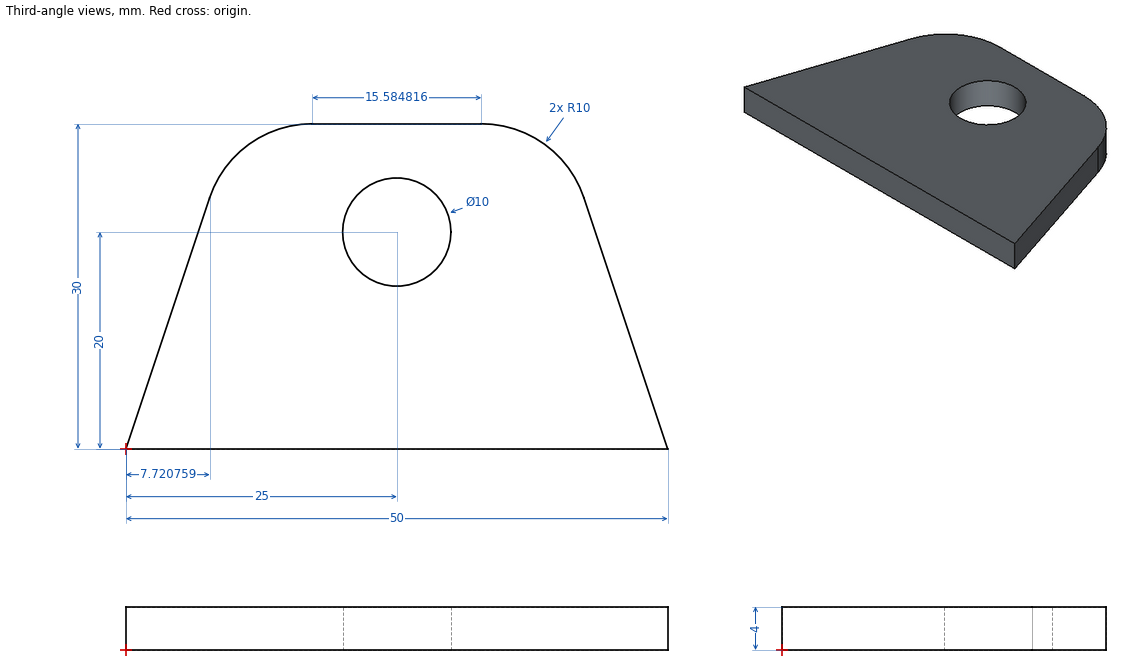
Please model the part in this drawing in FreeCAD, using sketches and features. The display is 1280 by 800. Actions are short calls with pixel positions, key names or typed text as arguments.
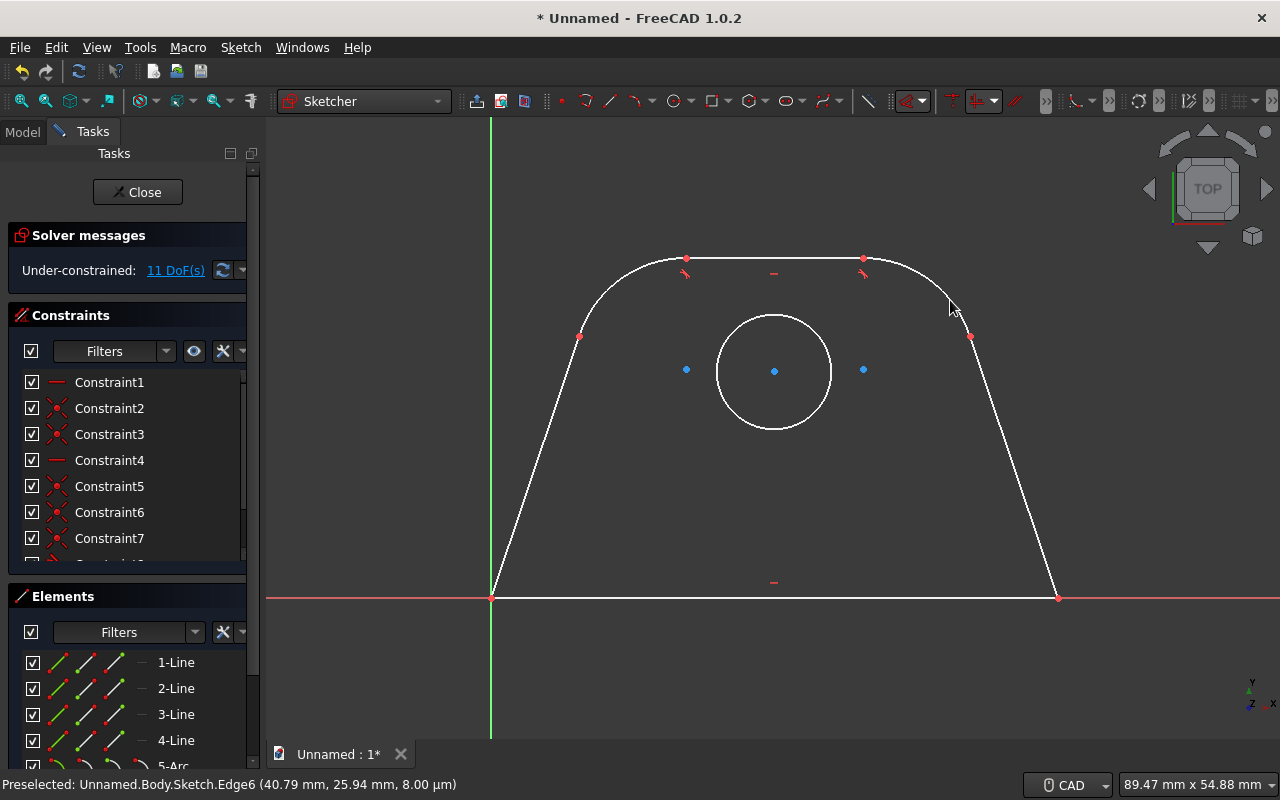
click(553, 415)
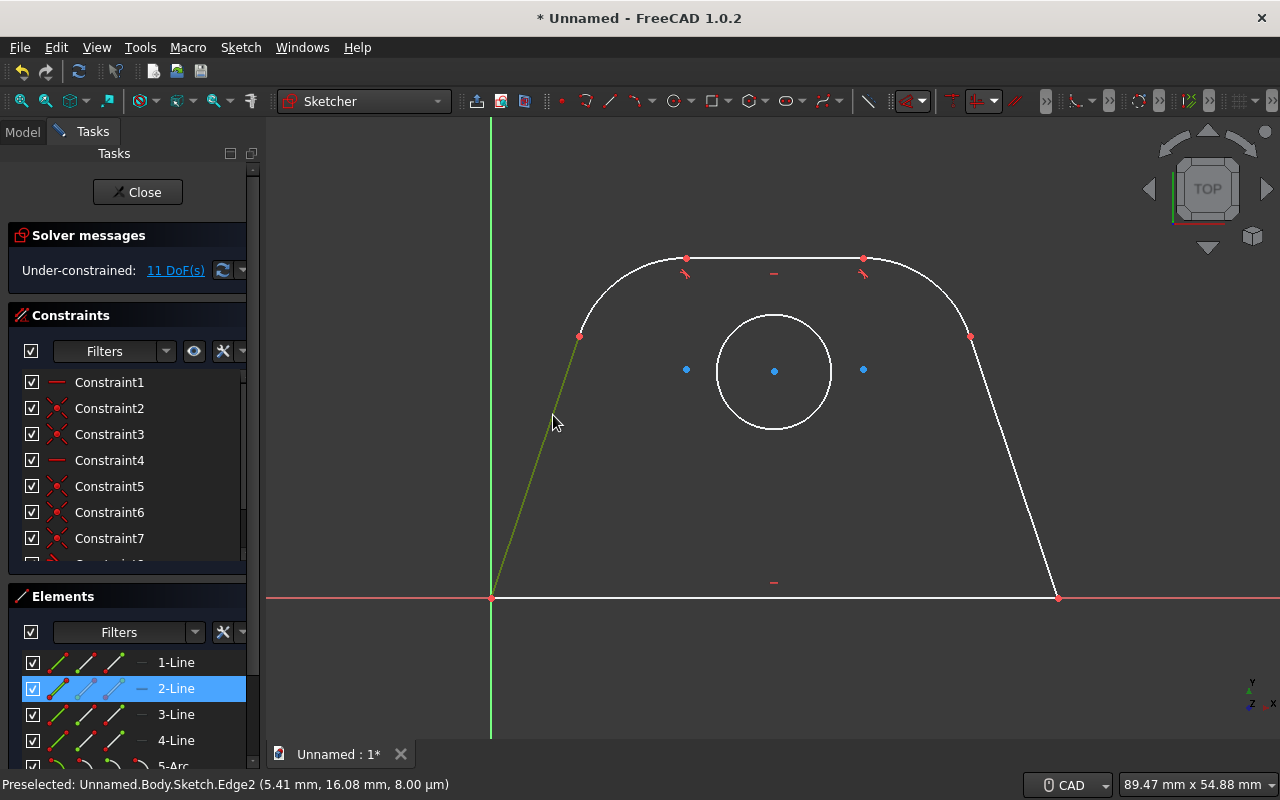
click(644, 266)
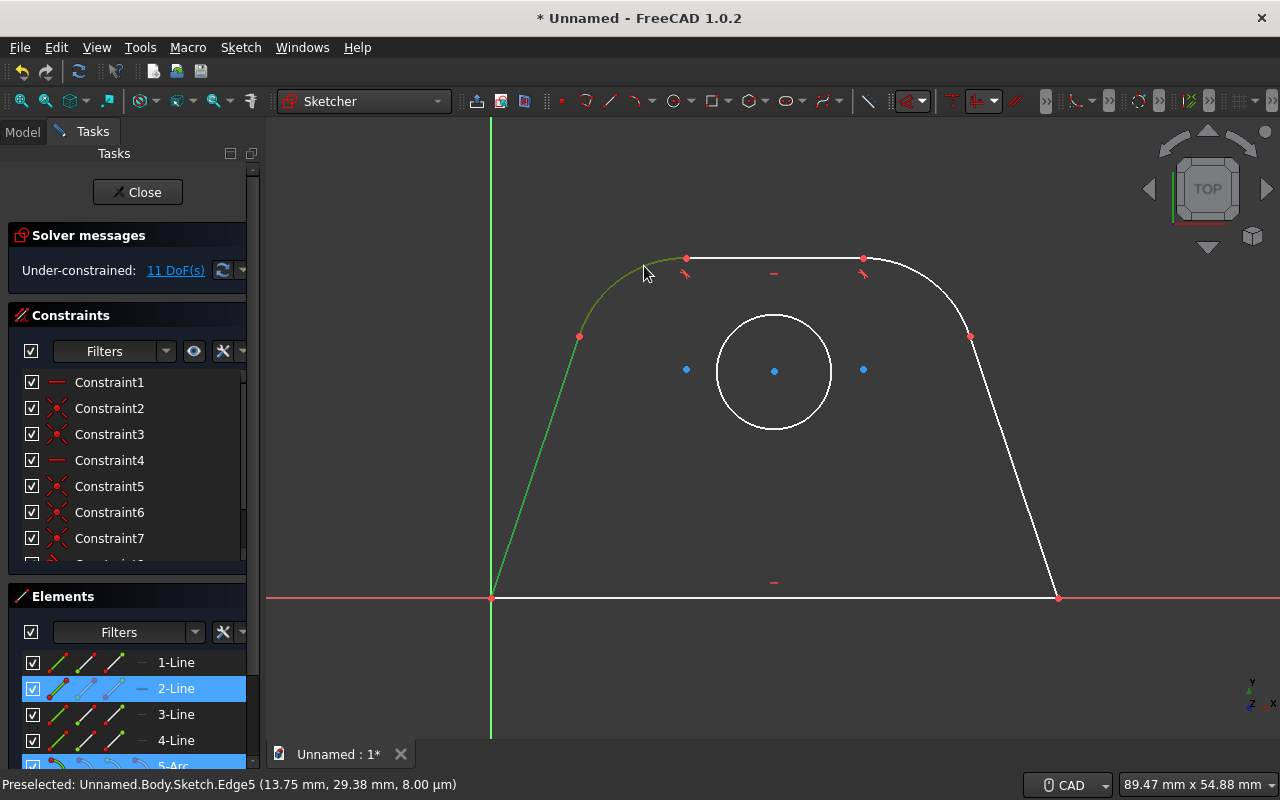
key(t)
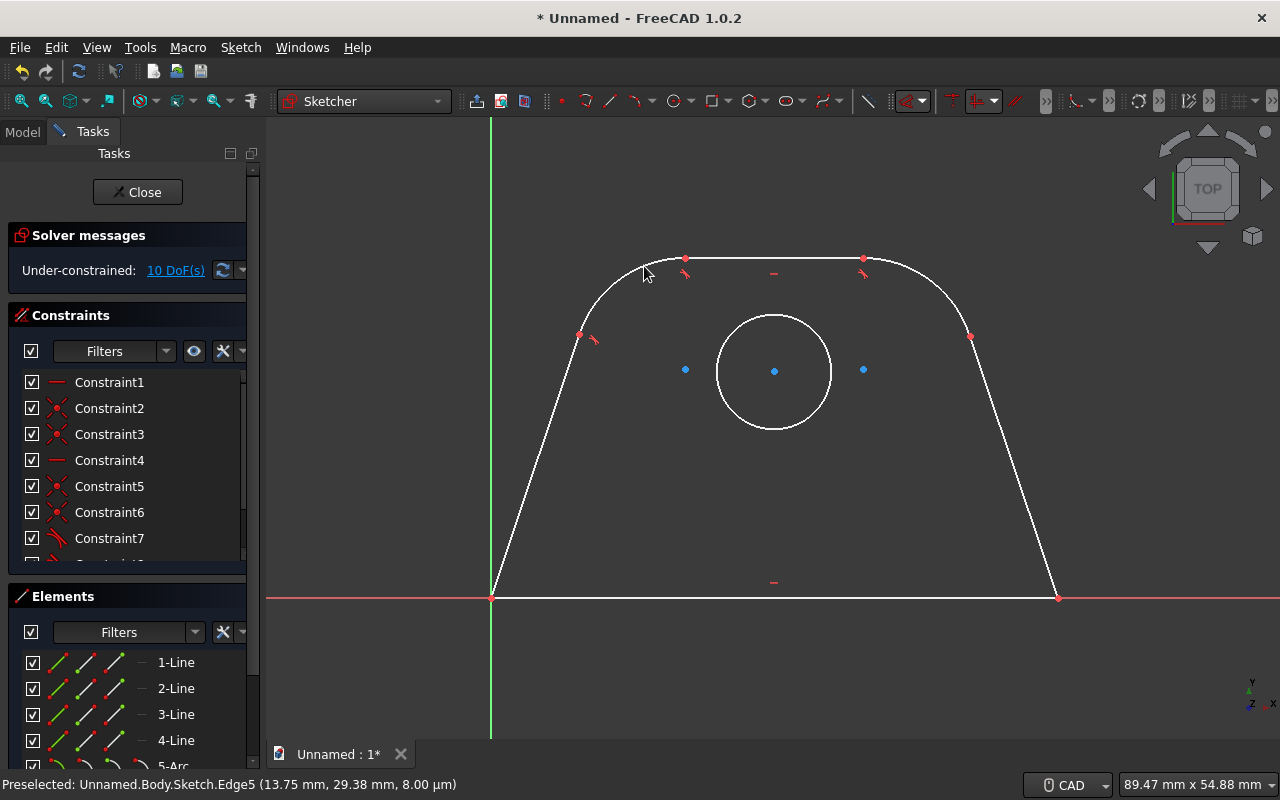
click(1032, 520)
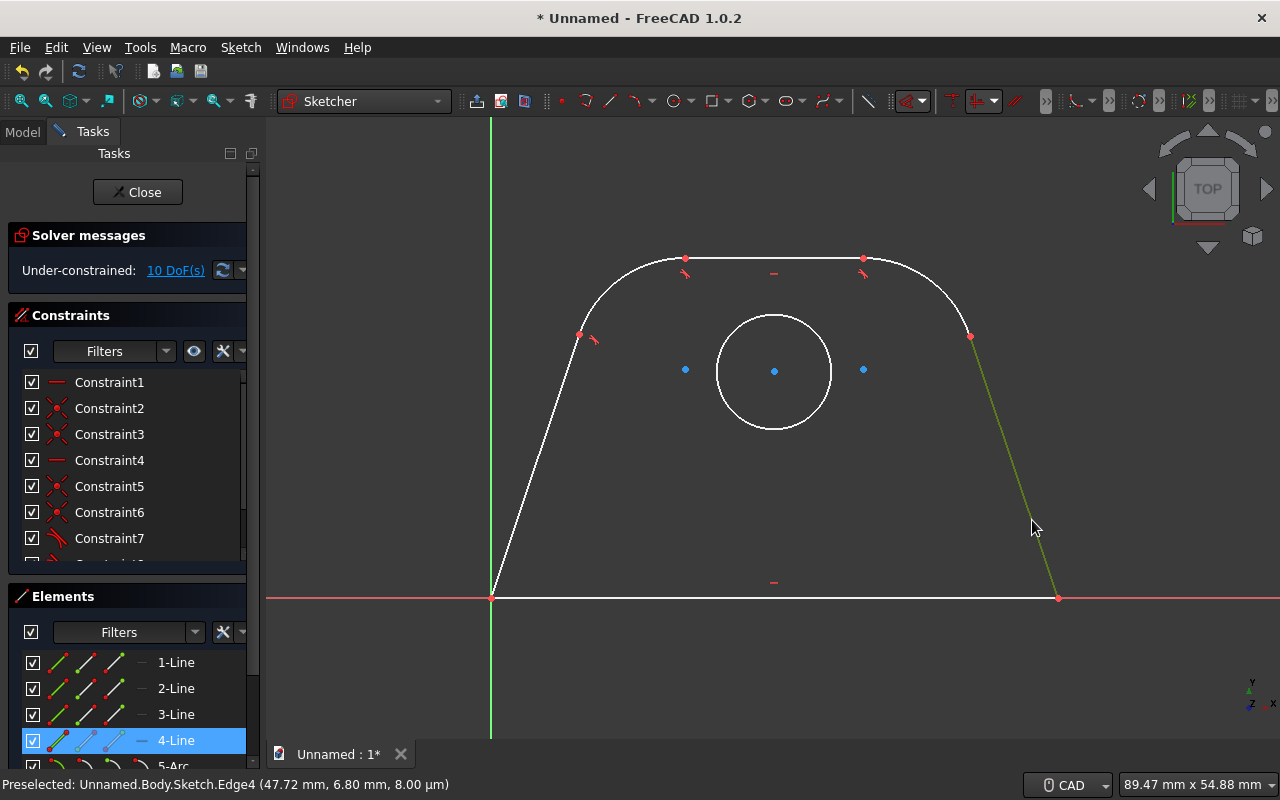
click(950, 300)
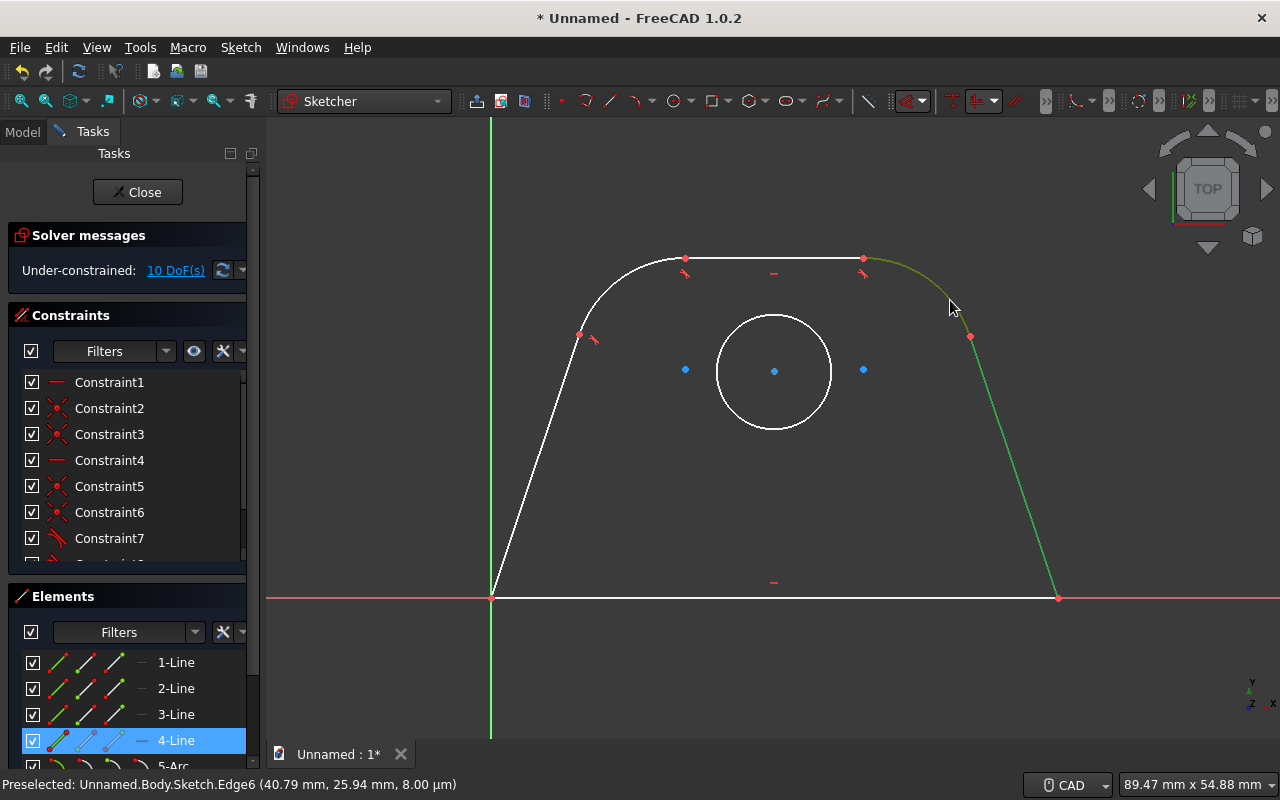
key(t)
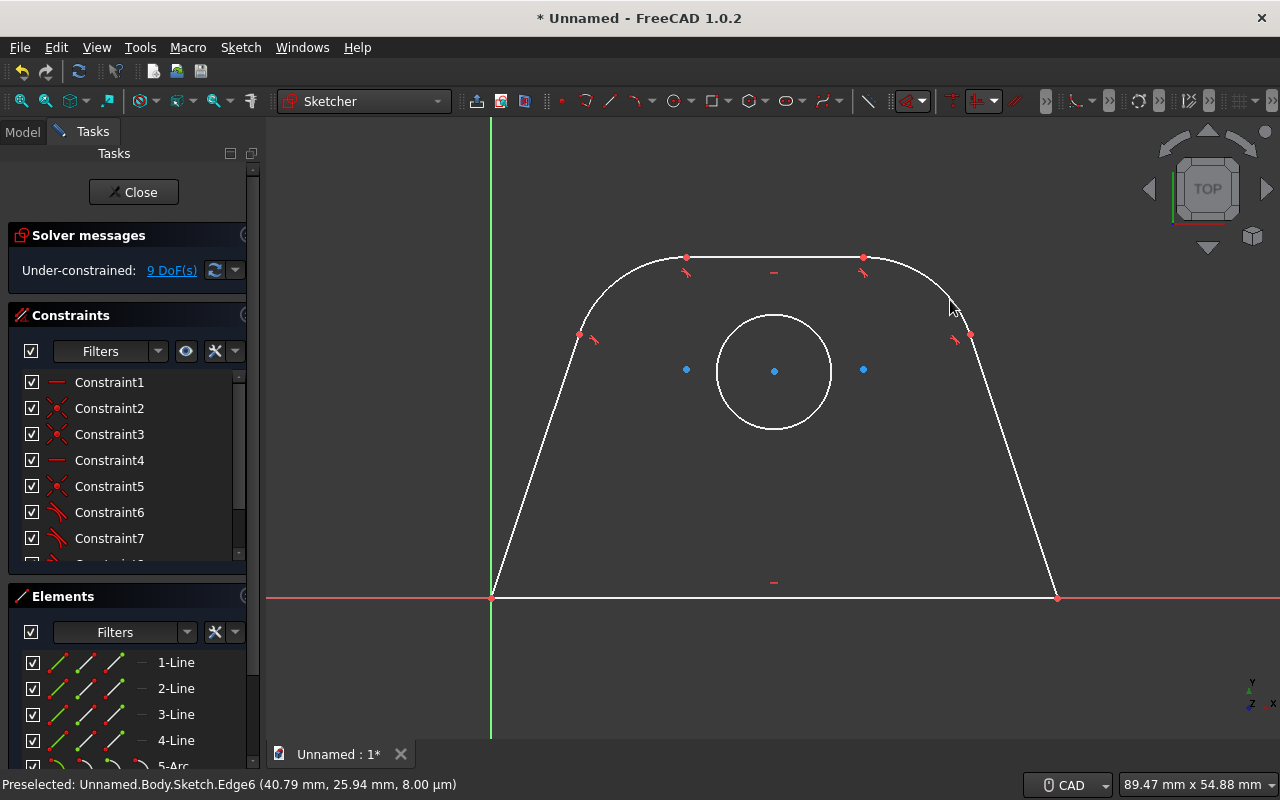
click(645, 265)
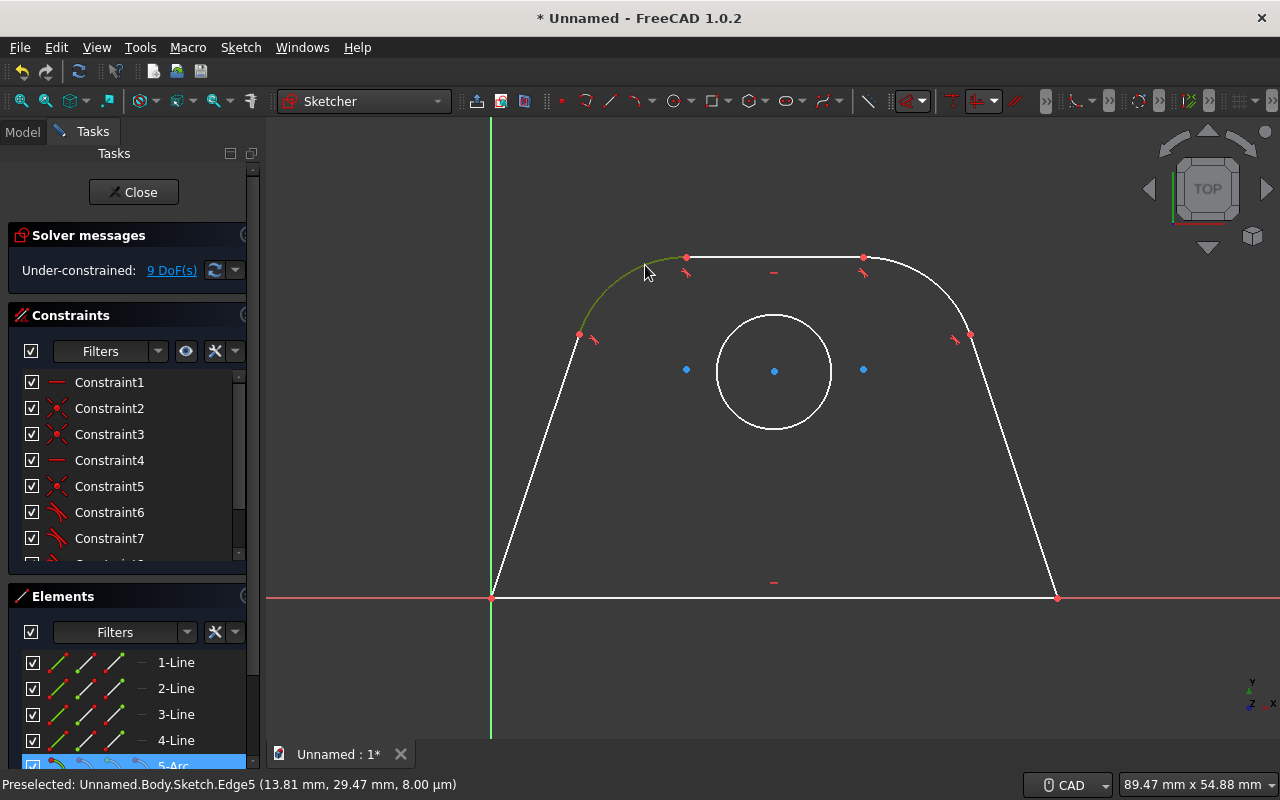
click(950, 298)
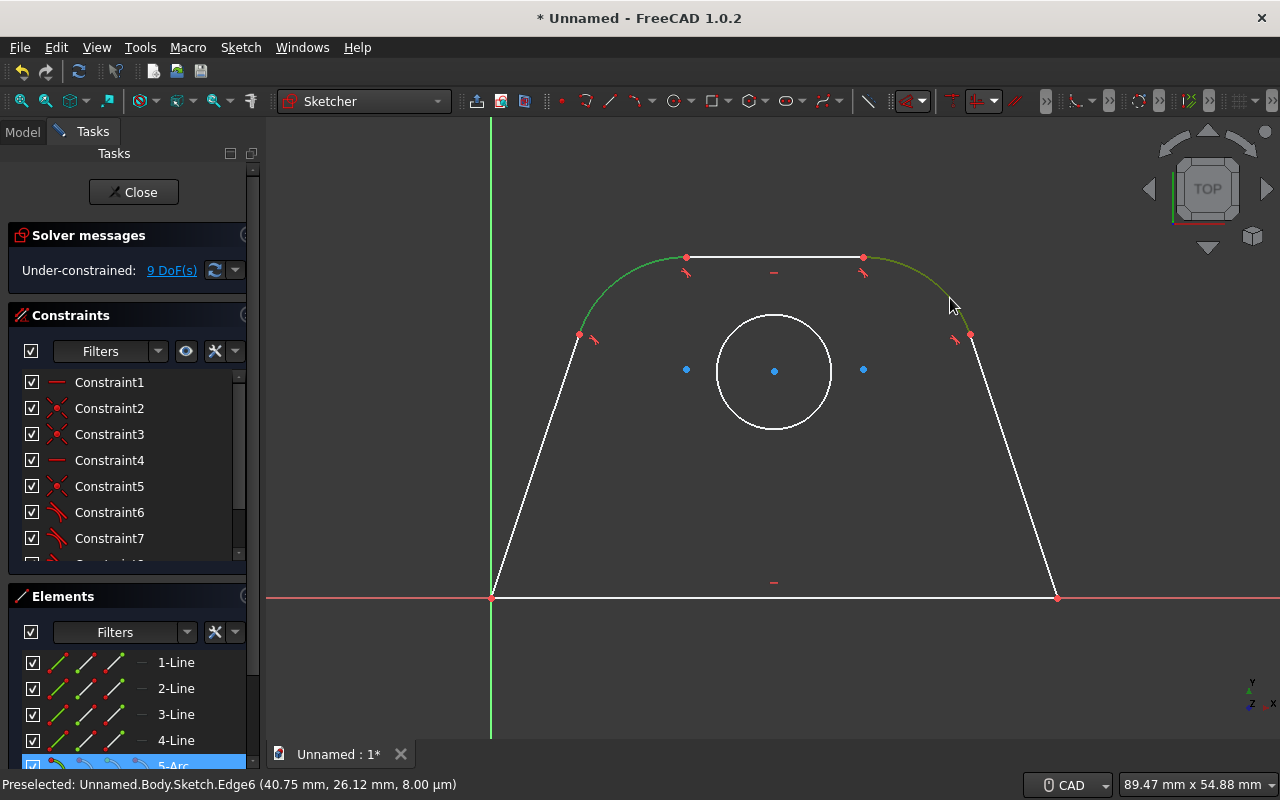
key(e)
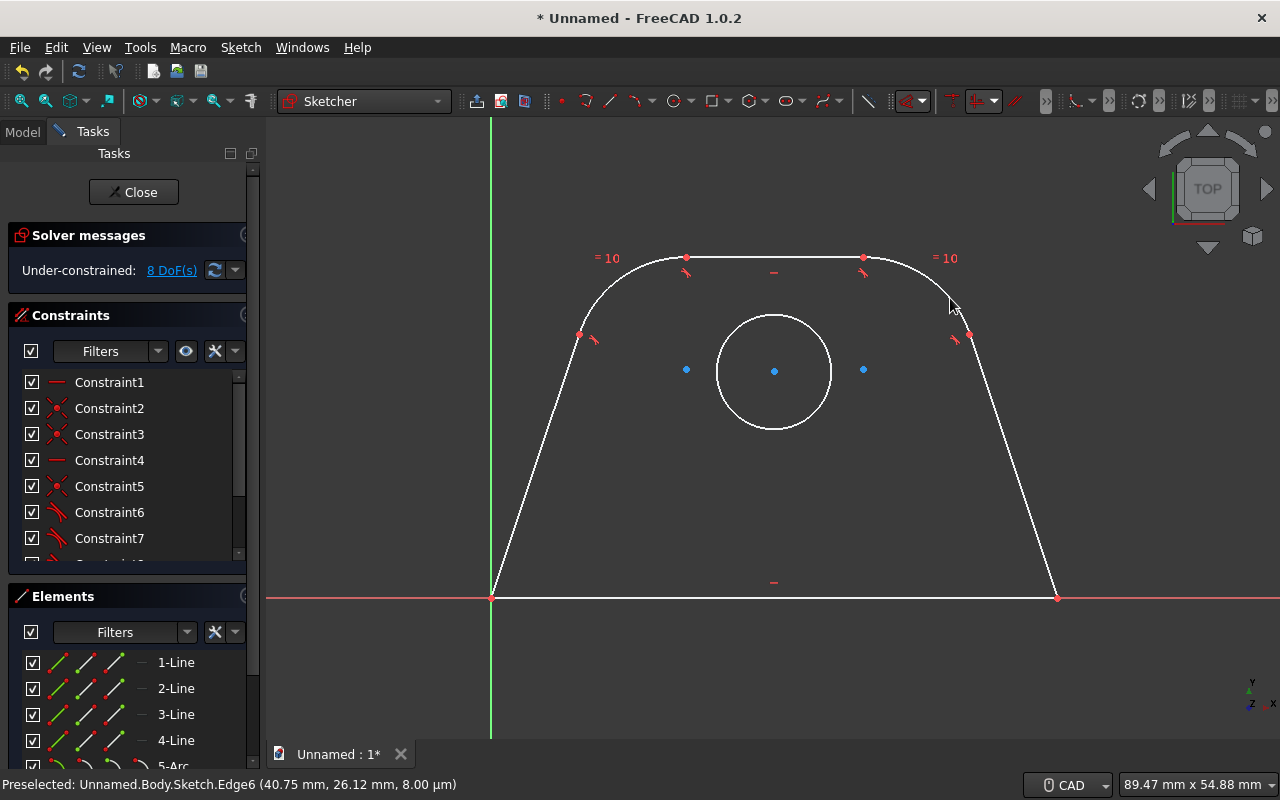
click(906, 102)